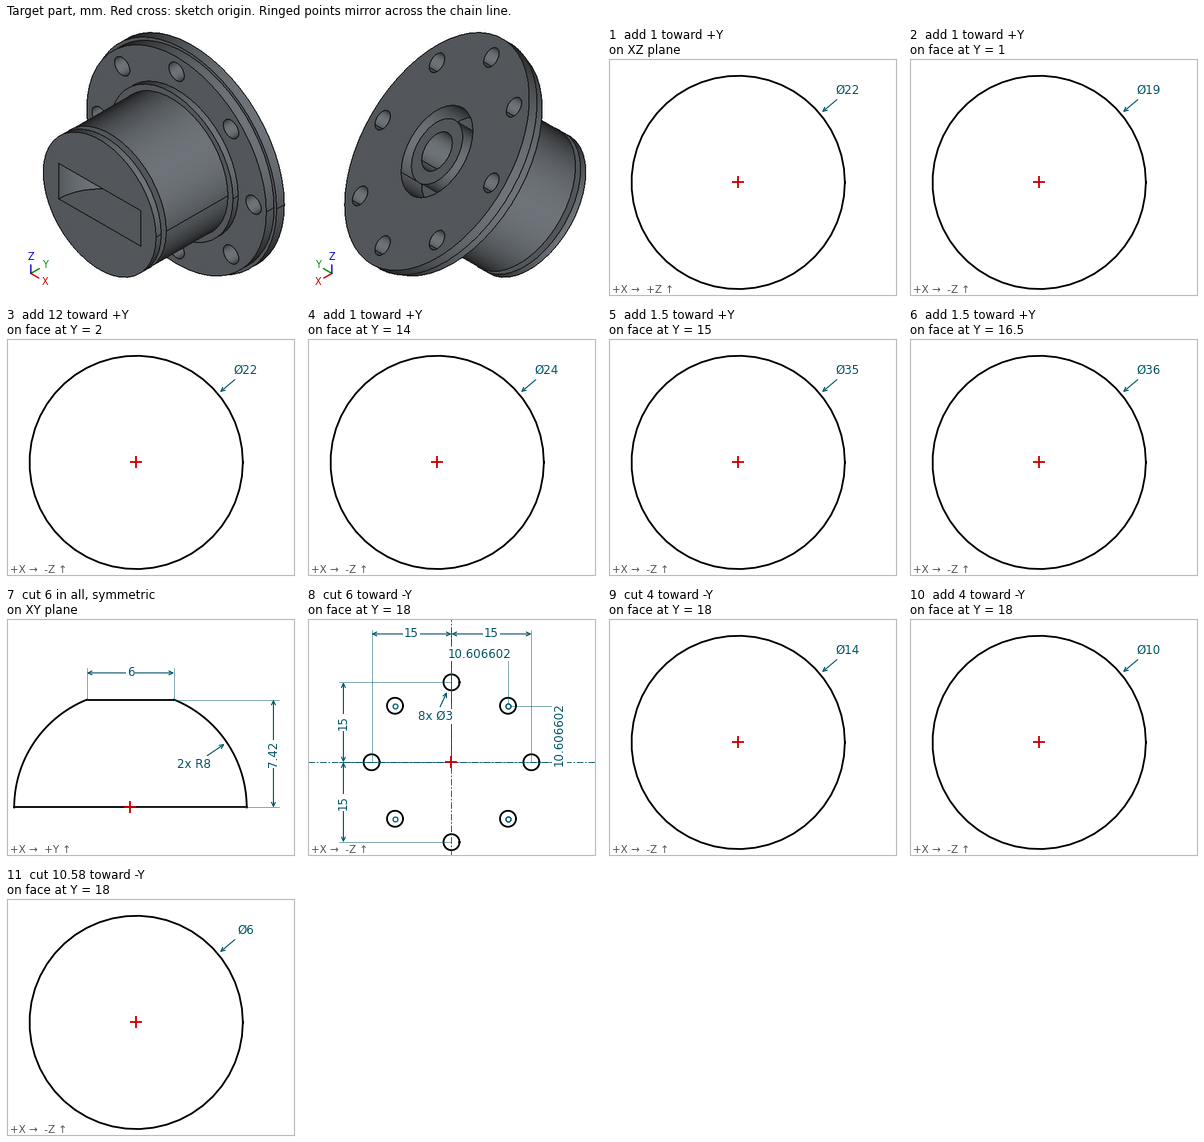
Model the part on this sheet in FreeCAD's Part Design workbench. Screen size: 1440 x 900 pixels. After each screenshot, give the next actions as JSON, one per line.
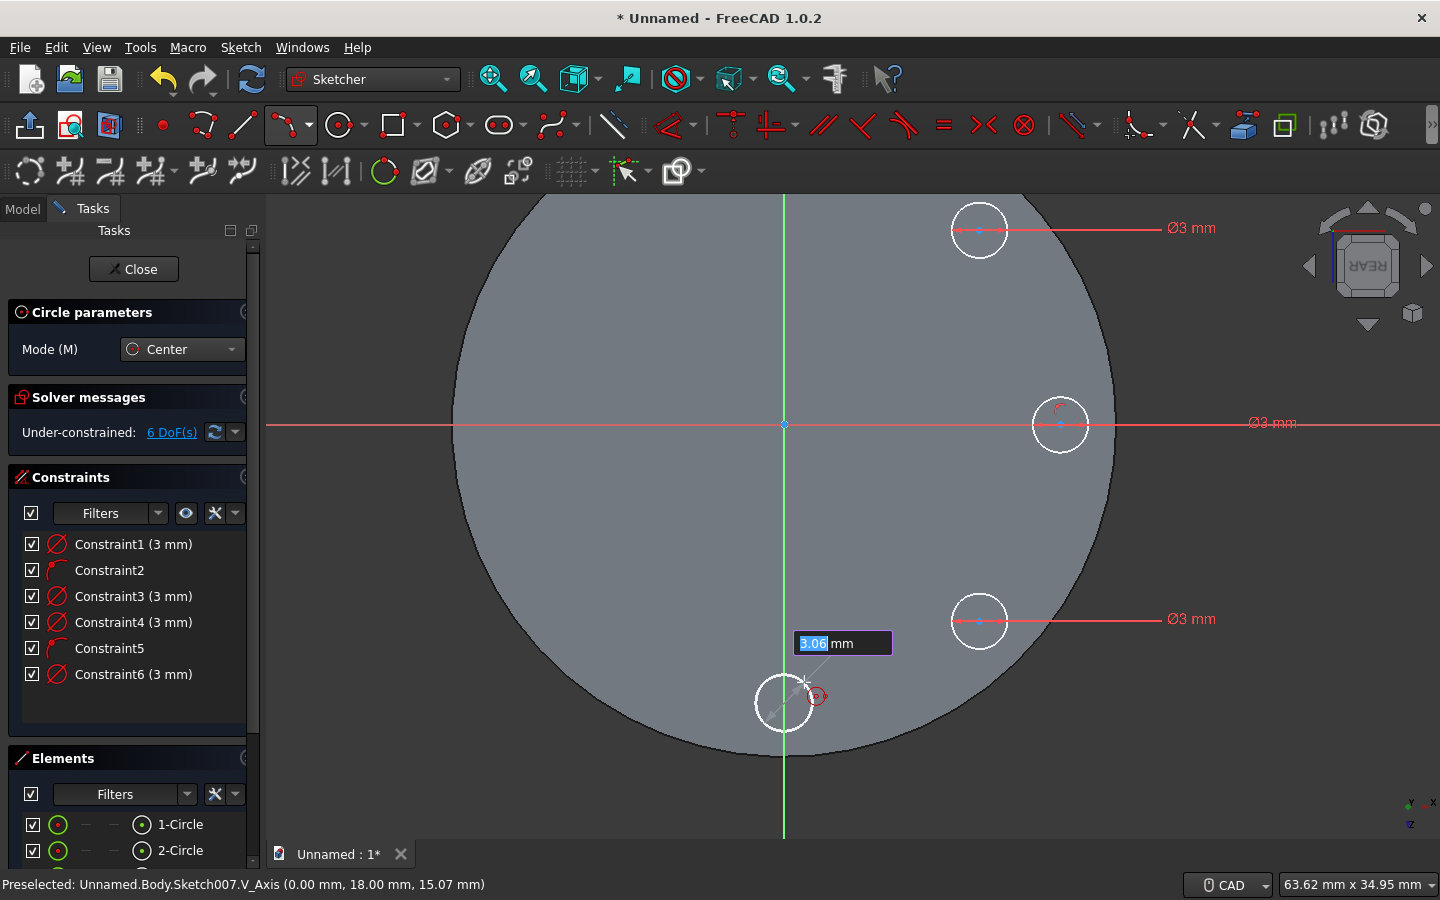
{"action": "type", "text": "3"}
{"action": "key", "text": "Return"}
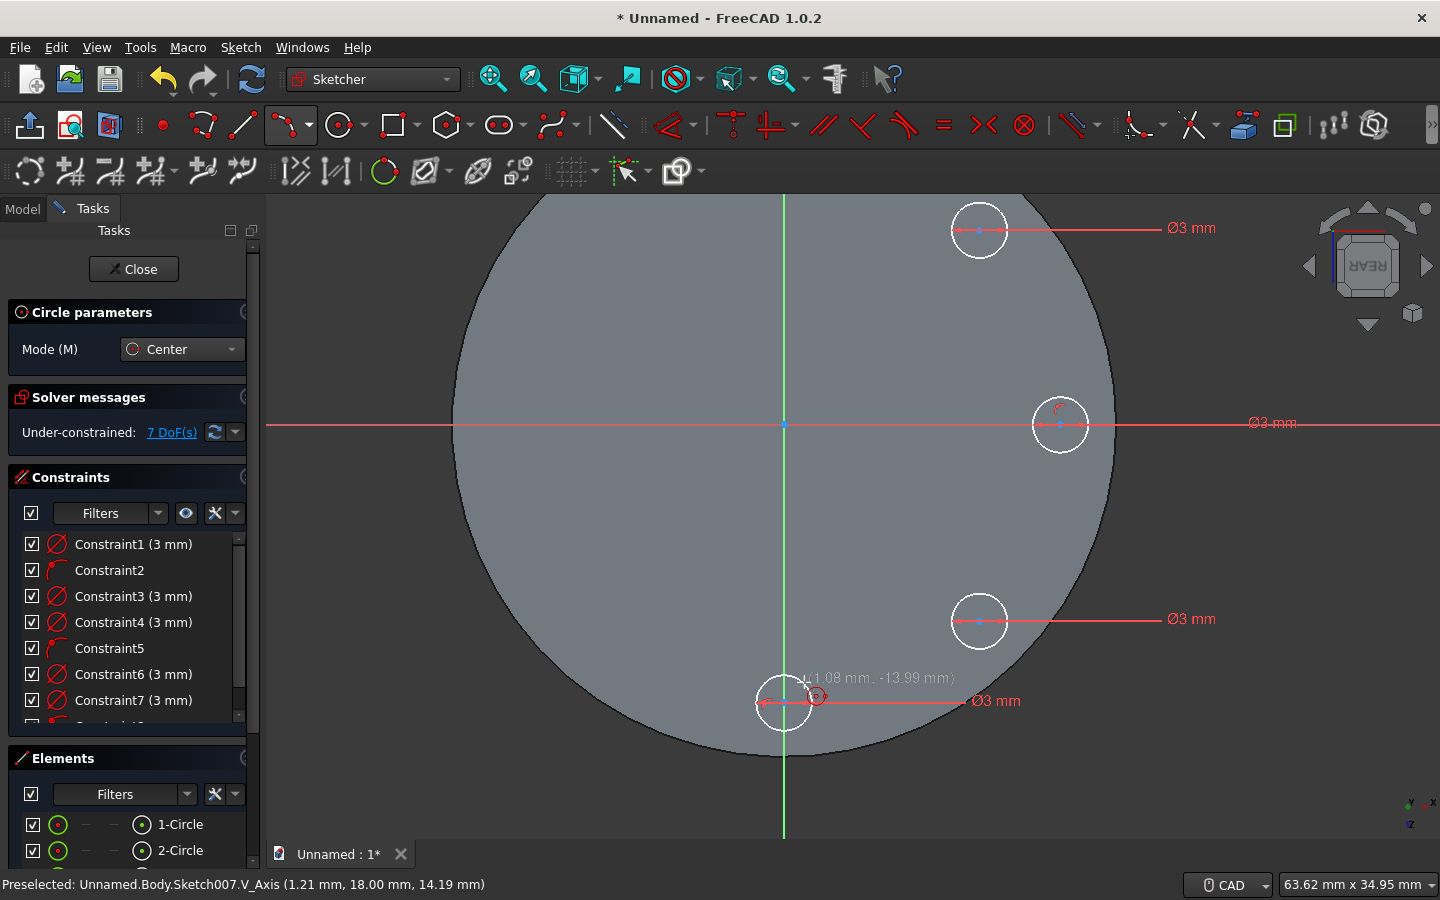
{"action": "left_click", "coordinate": [588, 621]}
{"action": "mouse_move", "coordinate": [608, 601]}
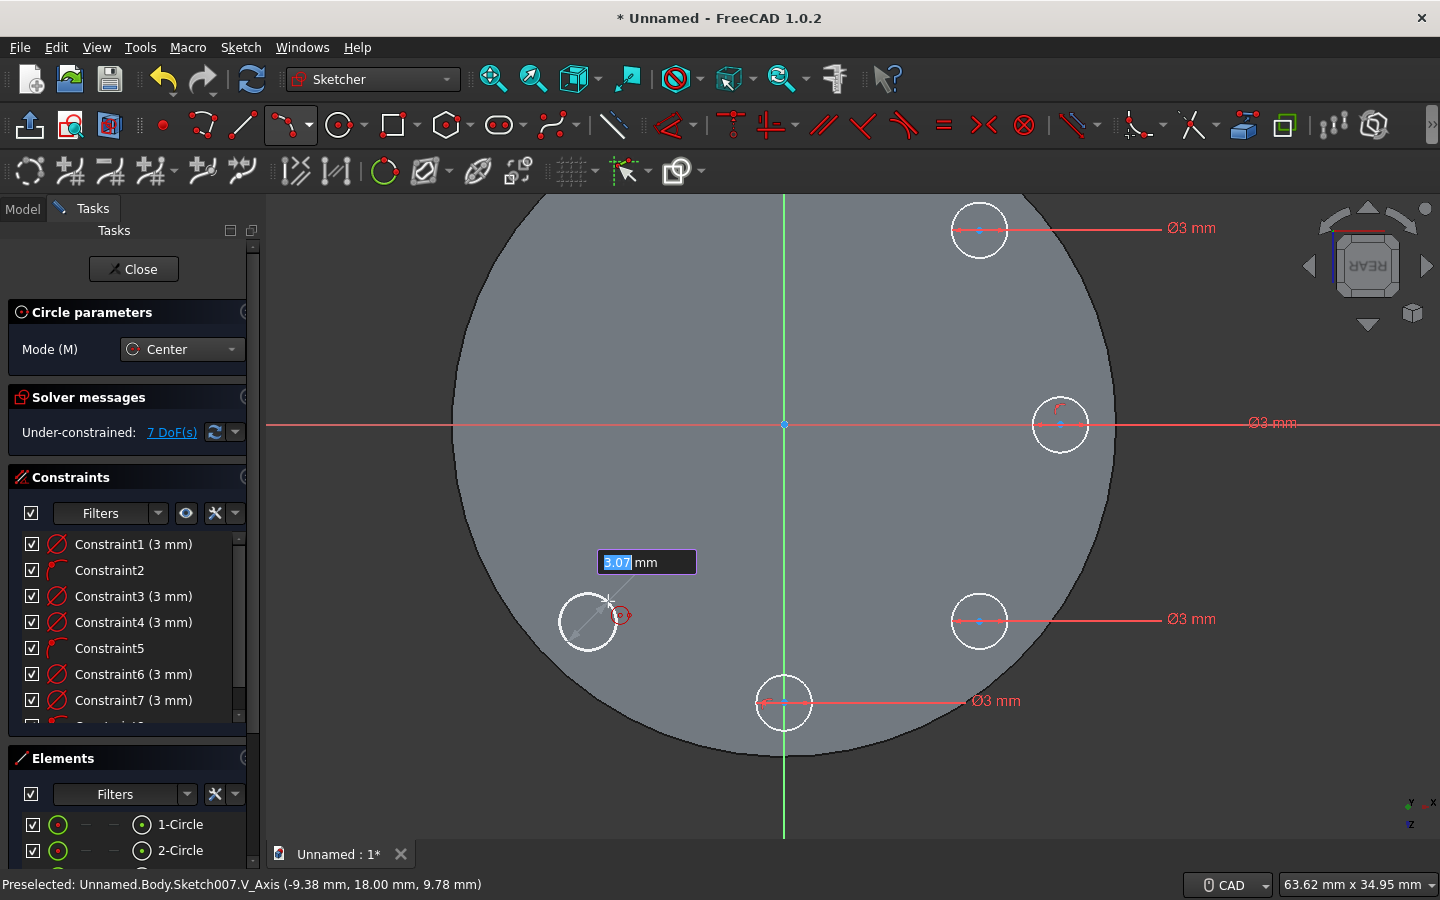
{"action": "type", "text": "3"}
{"action": "key", "text": "Return"}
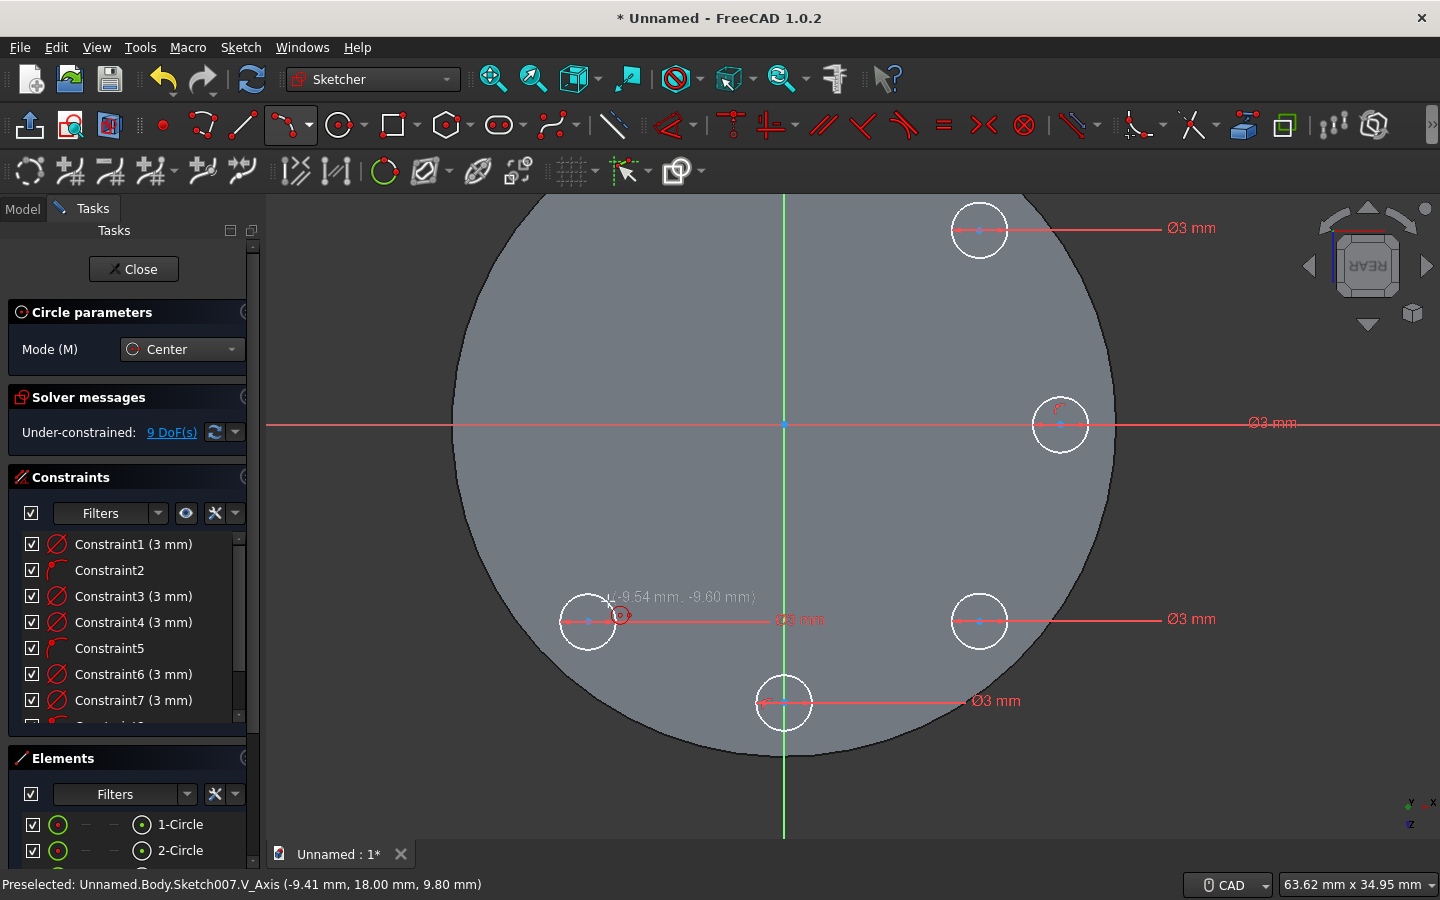
{"action": "left_click", "coordinate": [507, 425]}
{"action": "mouse_move", "coordinate": [527, 405]}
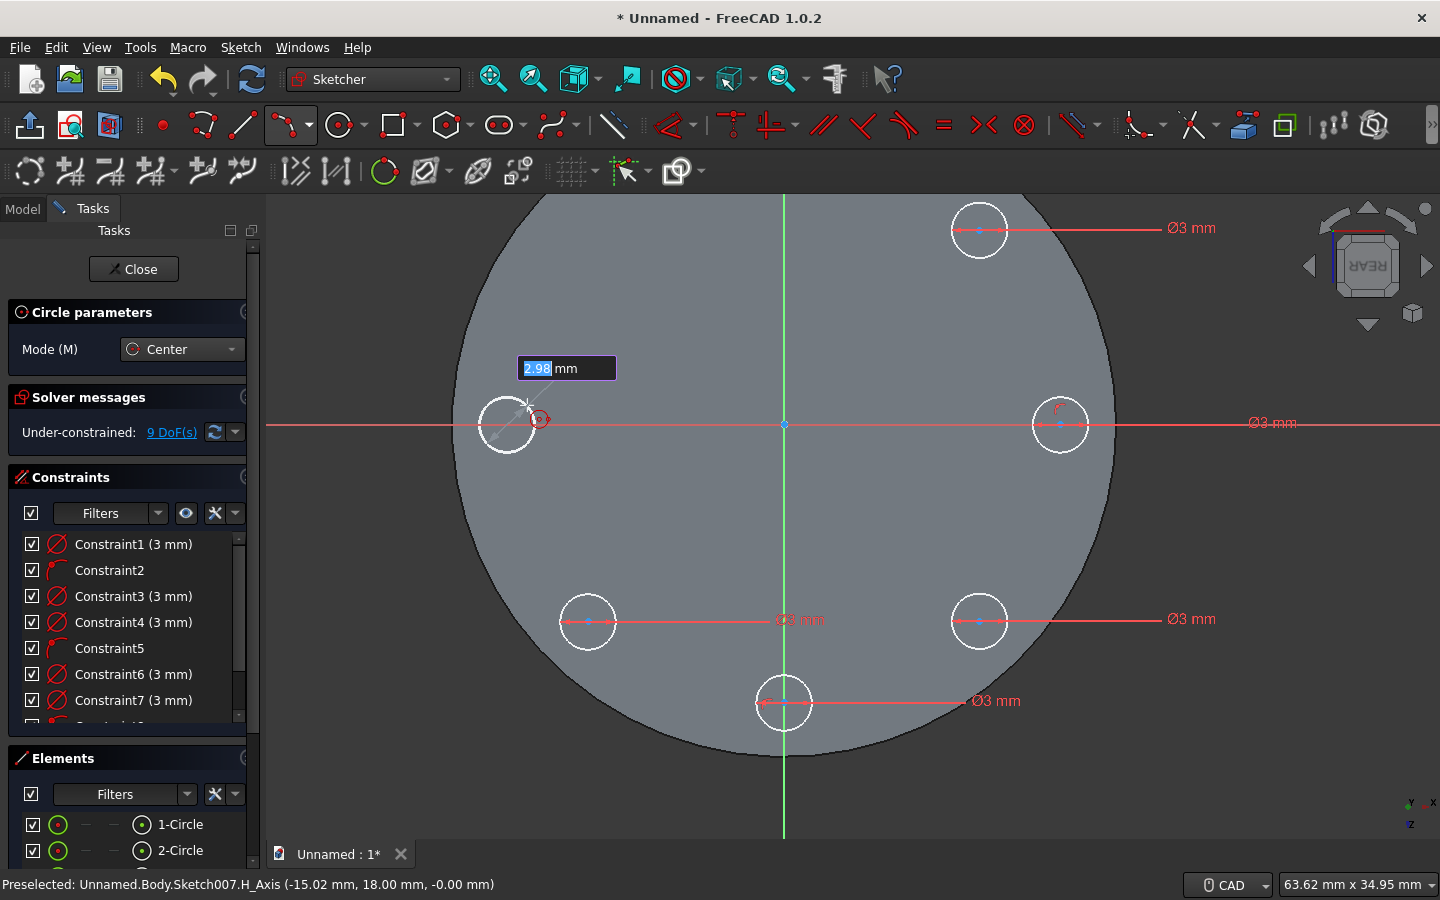
{"action": "type", "text": "3"}
{"action": "key", "text": "Return"}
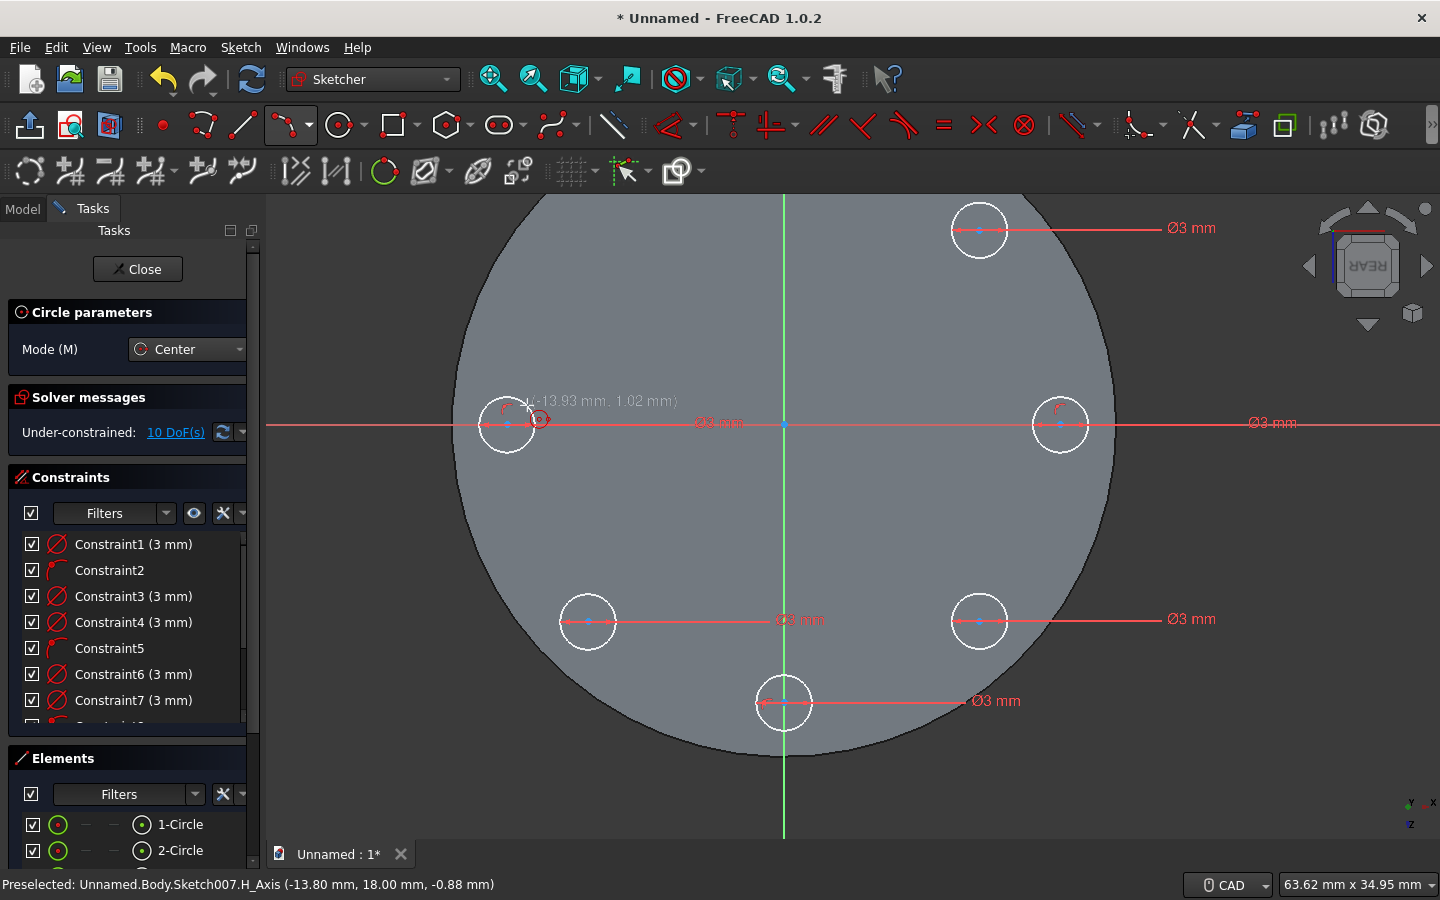
{"action": "left_click", "coordinate": [588, 229]}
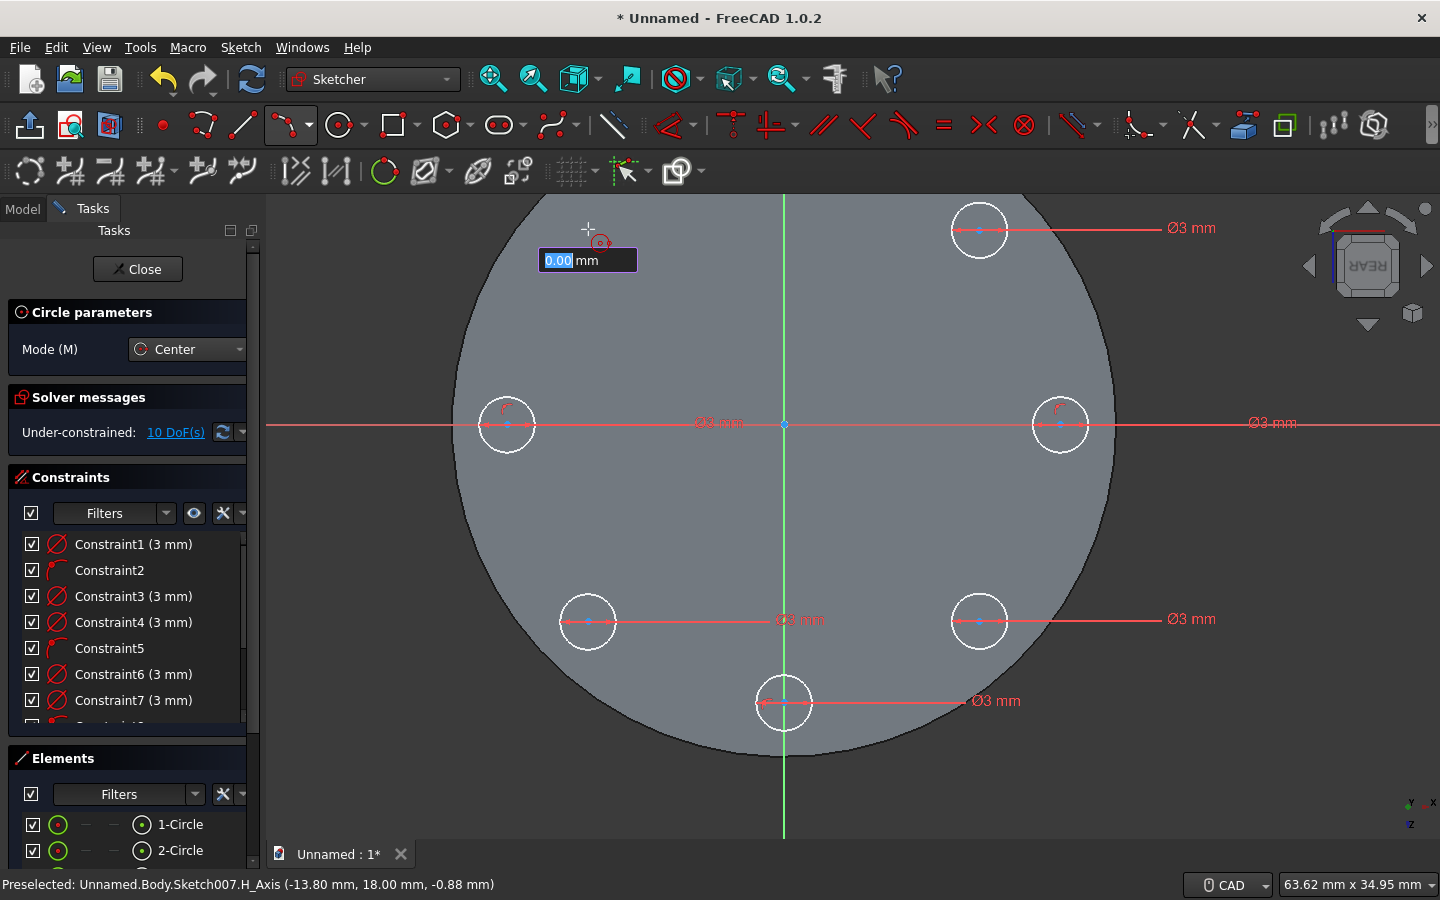
{"action": "scroll", "coordinate": [785, 703], "scroll_direction": "down", "scroll_amount": 2}
{"action": "mouse_move", "coordinate": [666, 373]}